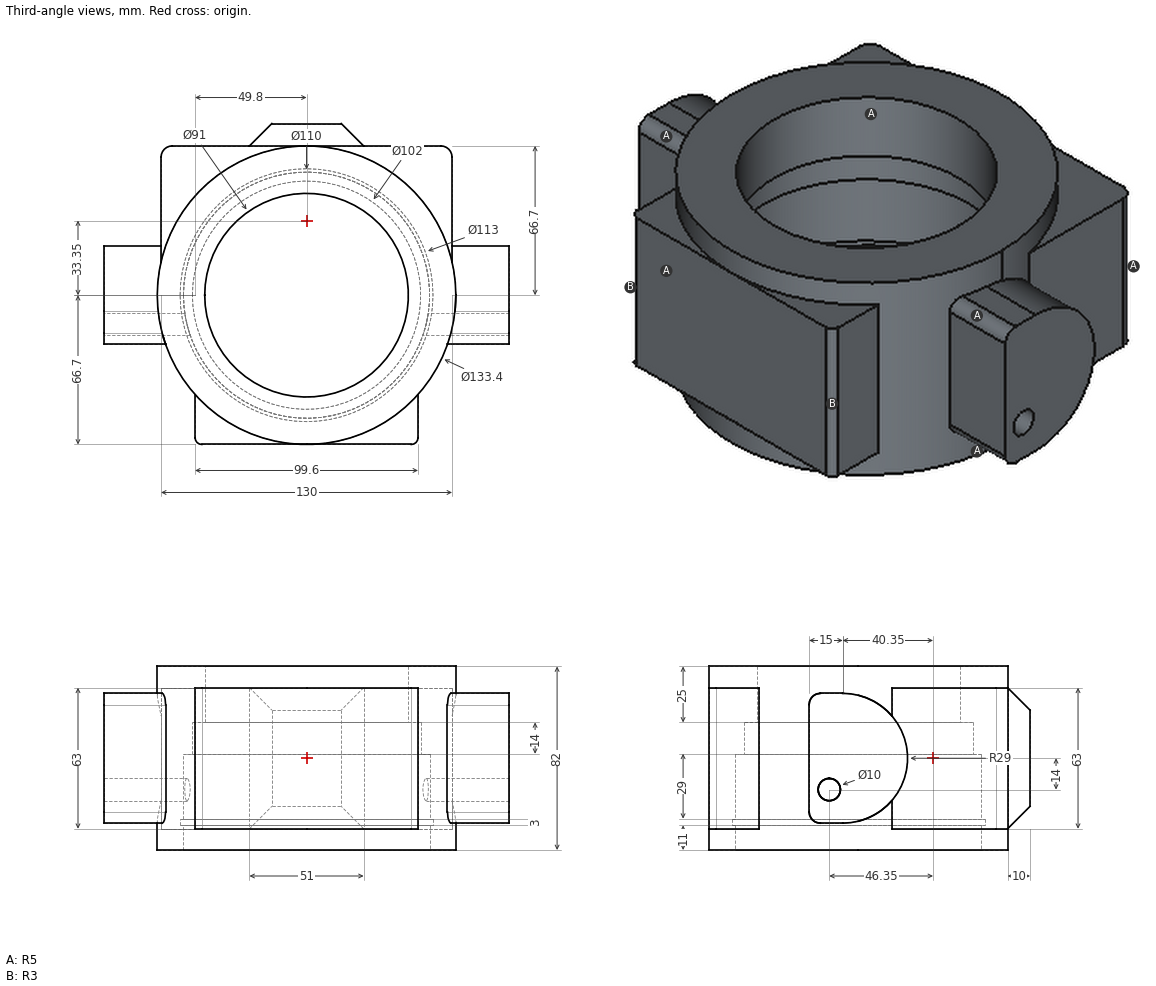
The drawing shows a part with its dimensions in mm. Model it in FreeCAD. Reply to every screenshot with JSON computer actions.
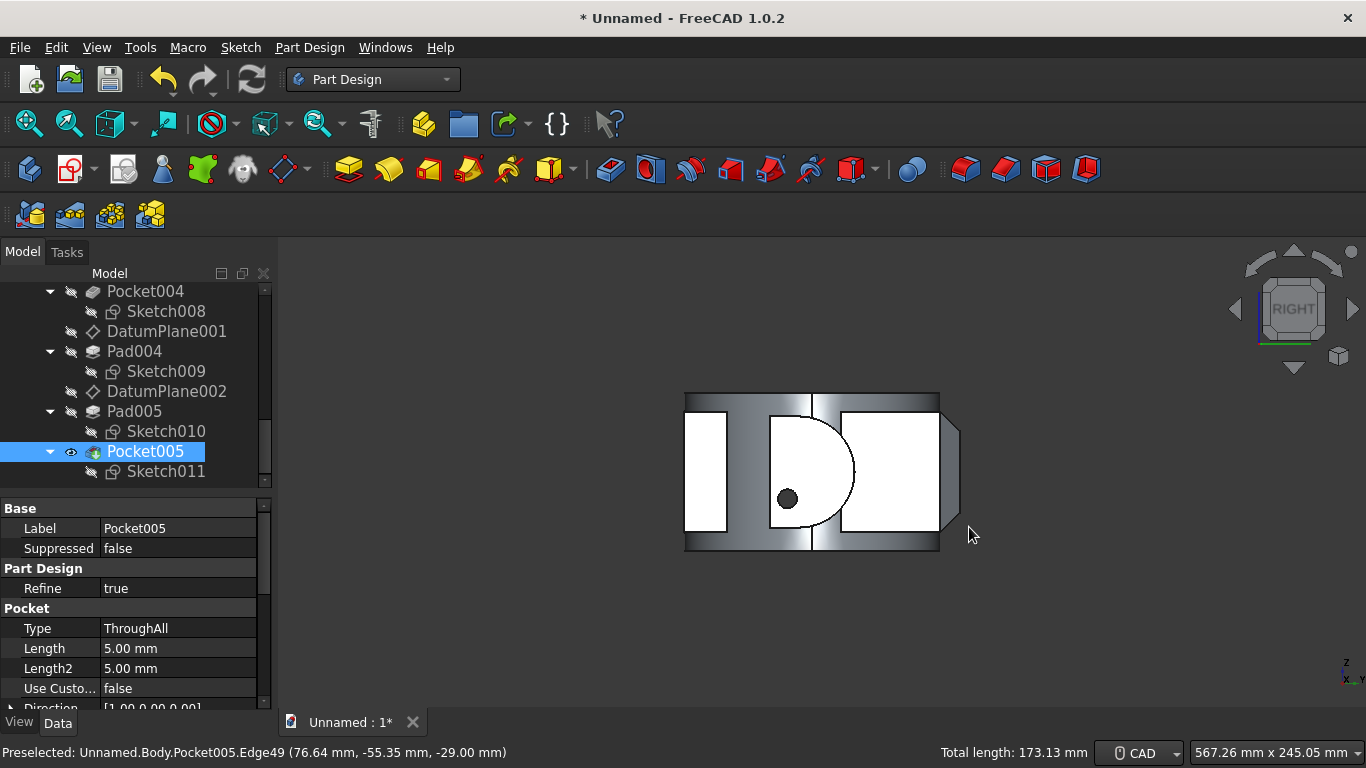
{"action": "key", "text": "v f"}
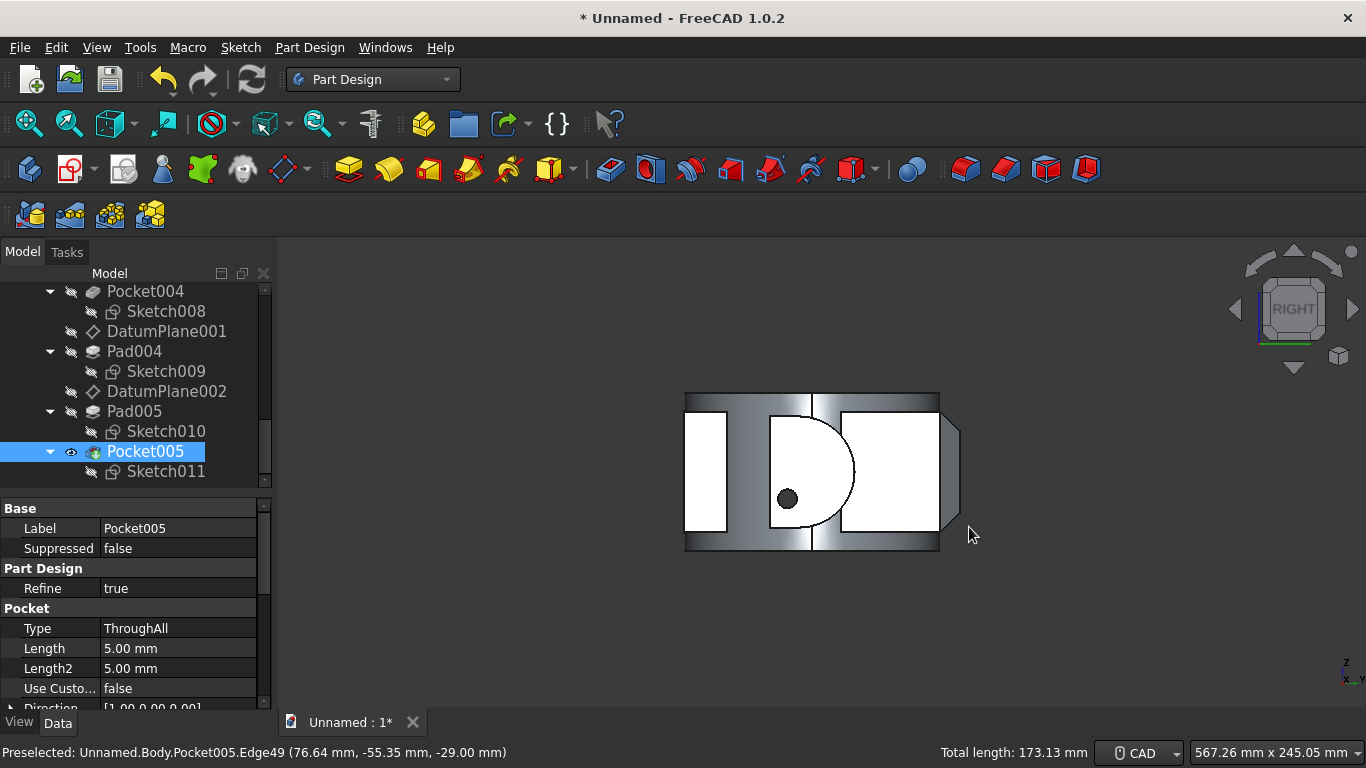
{"action": "left_click", "coordinate": [940, 471], "text": "ctrl"}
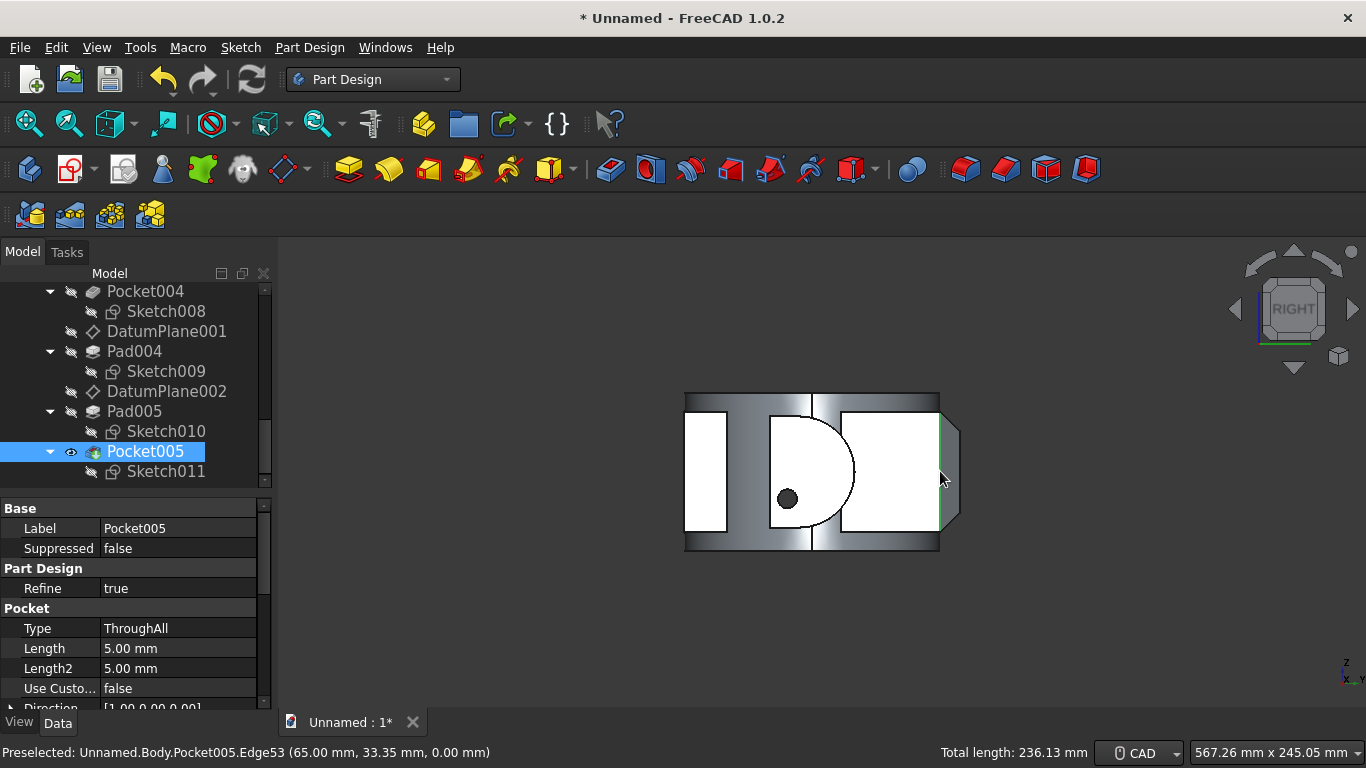
{"action": "left_click", "coordinate": [966, 170]}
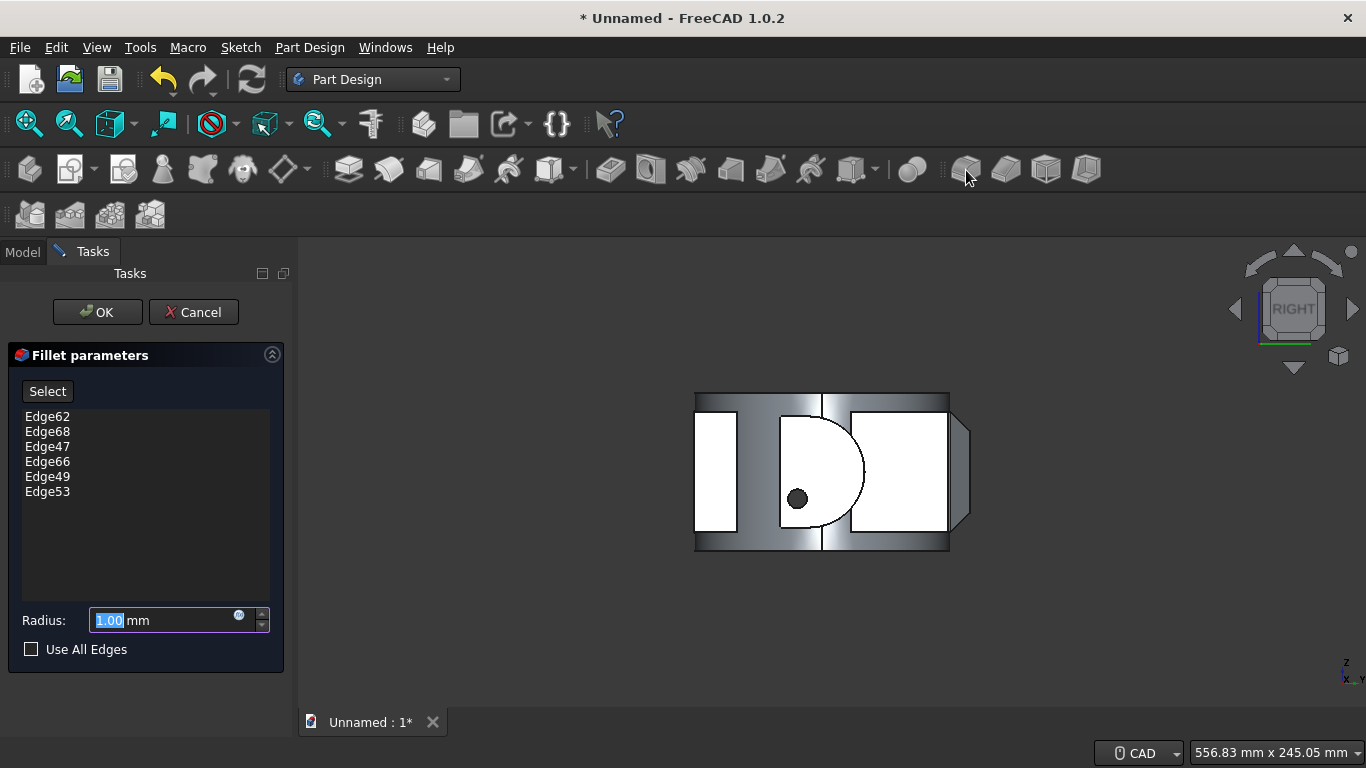
{"action": "type", "text": "5"}
{"action": "key", "text": "Tab"}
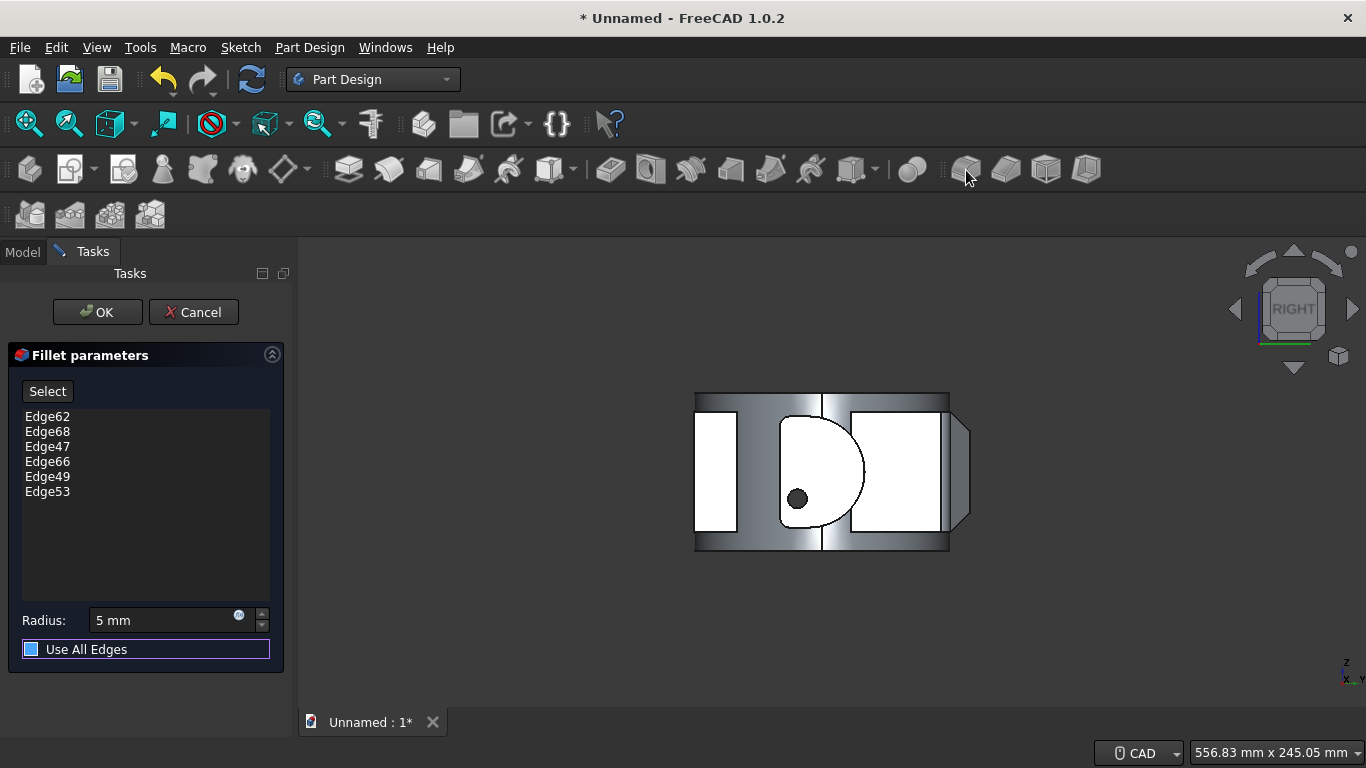
{"action": "left_click", "coordinate": [98, 312]}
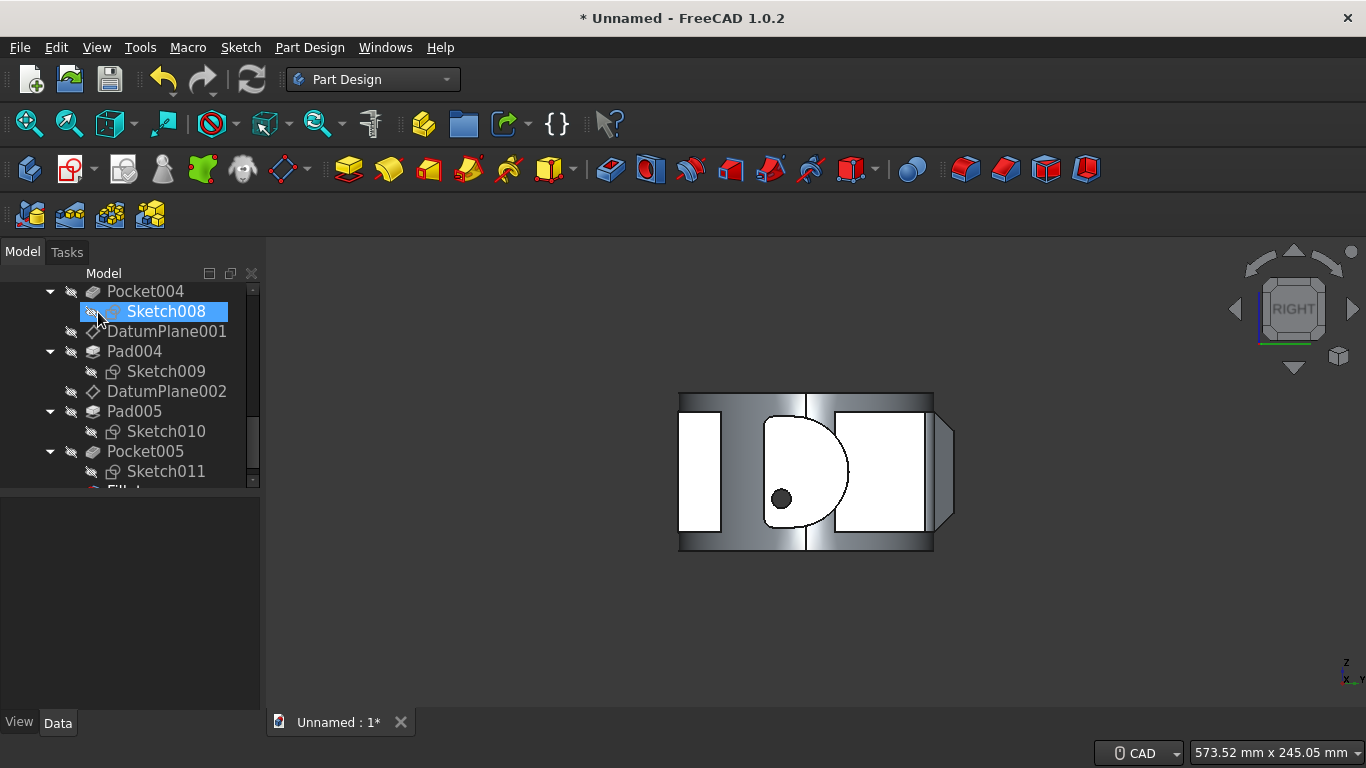
{"action": "key", "text": "v f"}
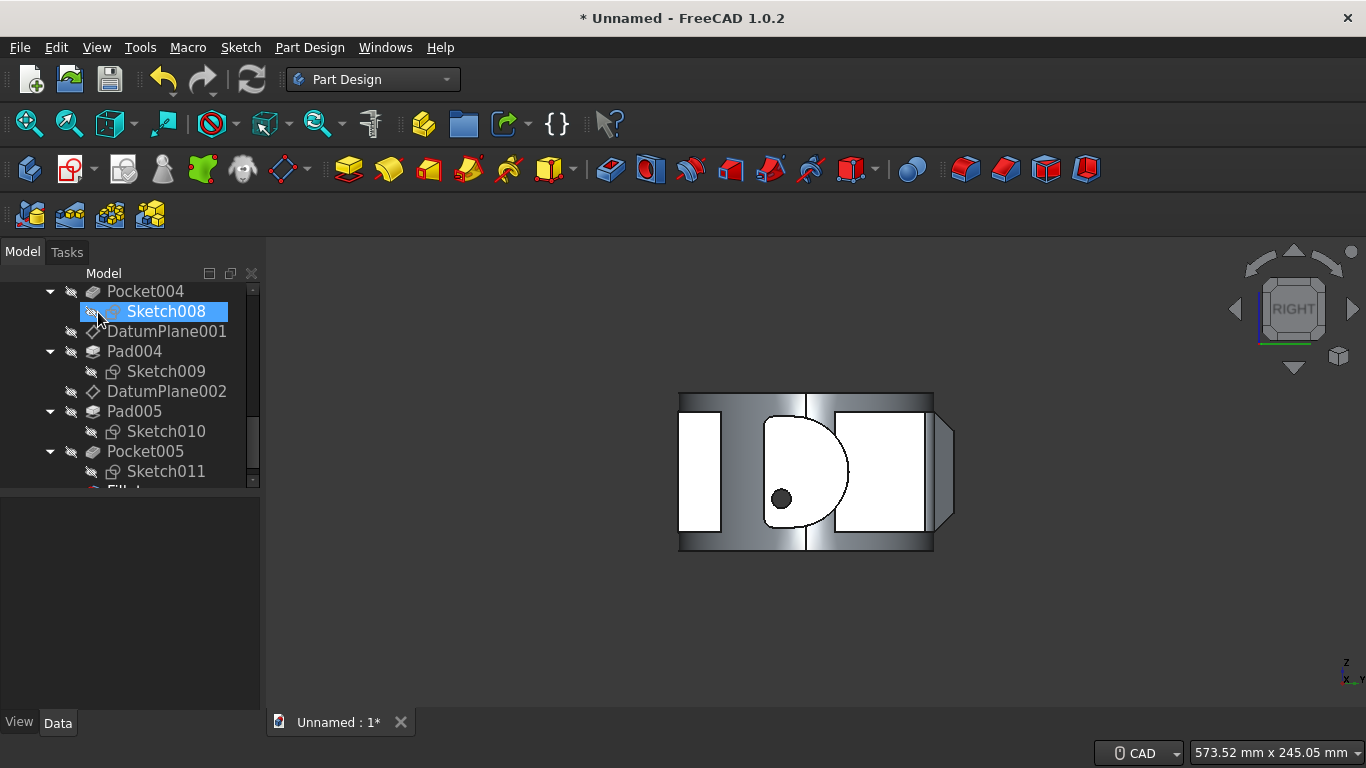
{"action": "left_click", "coordinate": [678, 471]}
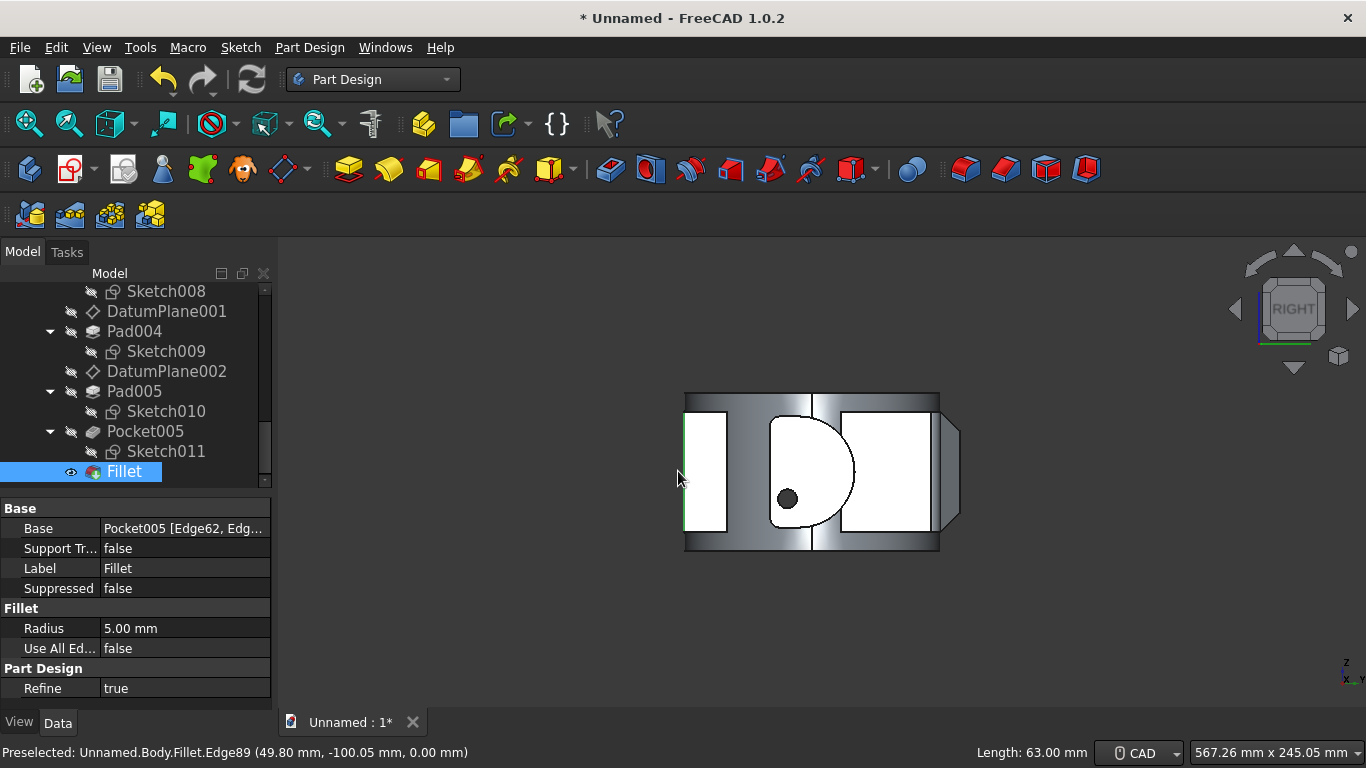
{"action": "key", "text": "0"}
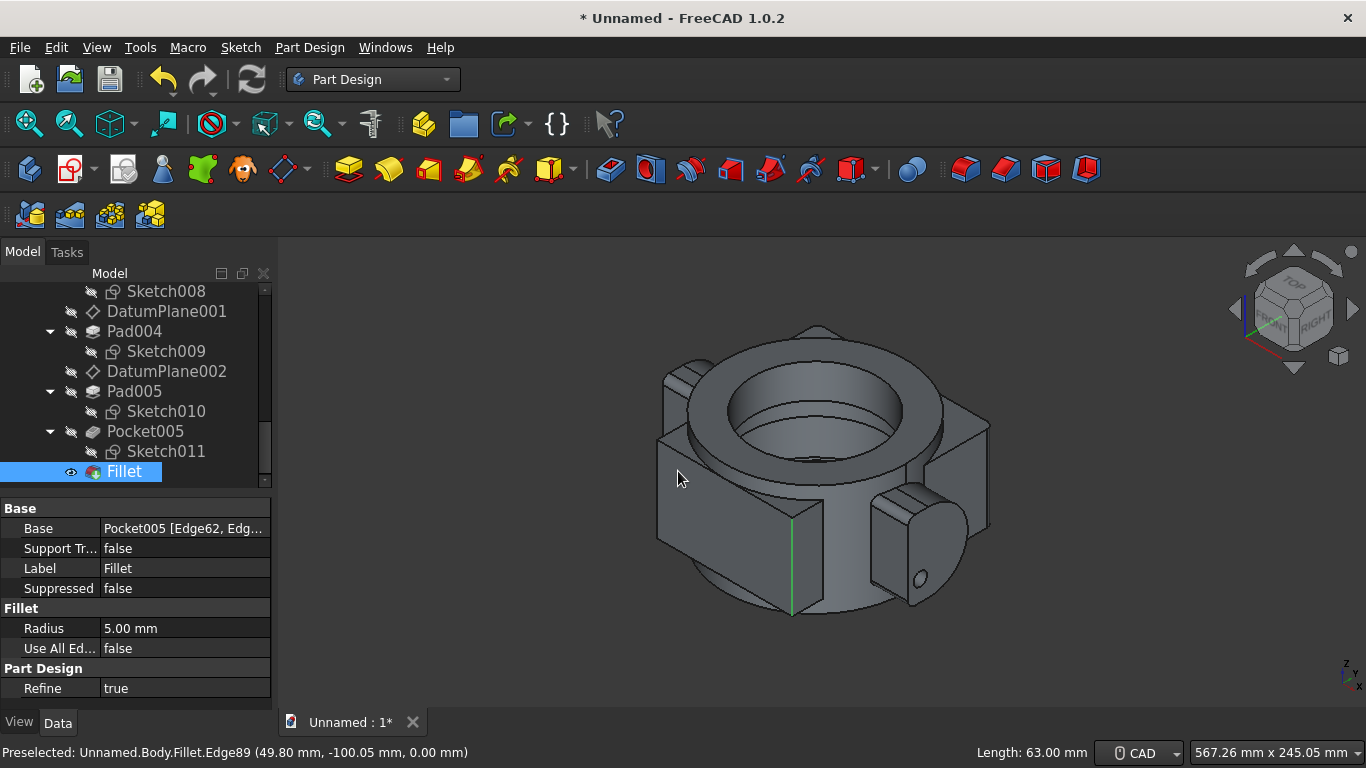
{"action": "key", "text": "2"}